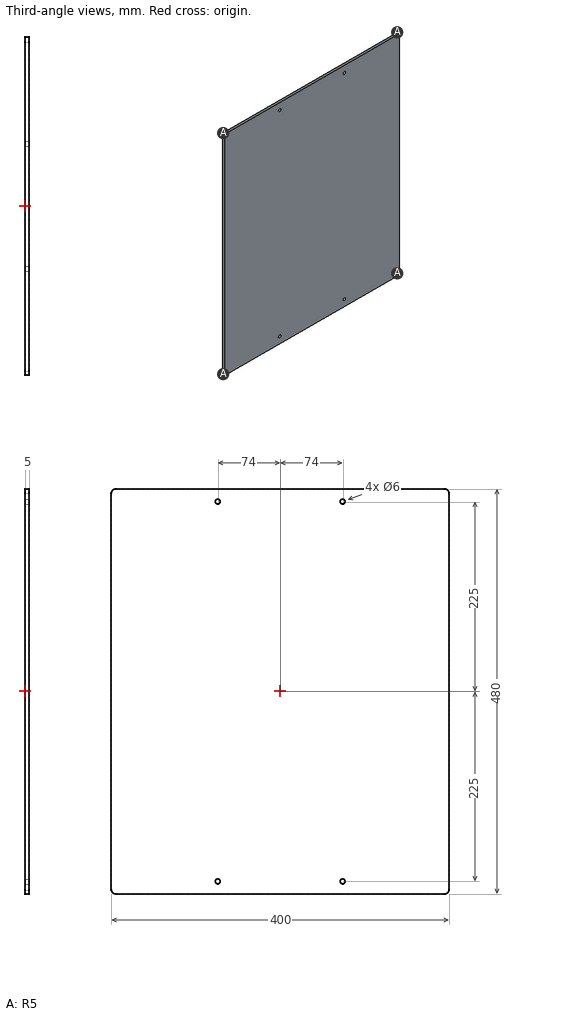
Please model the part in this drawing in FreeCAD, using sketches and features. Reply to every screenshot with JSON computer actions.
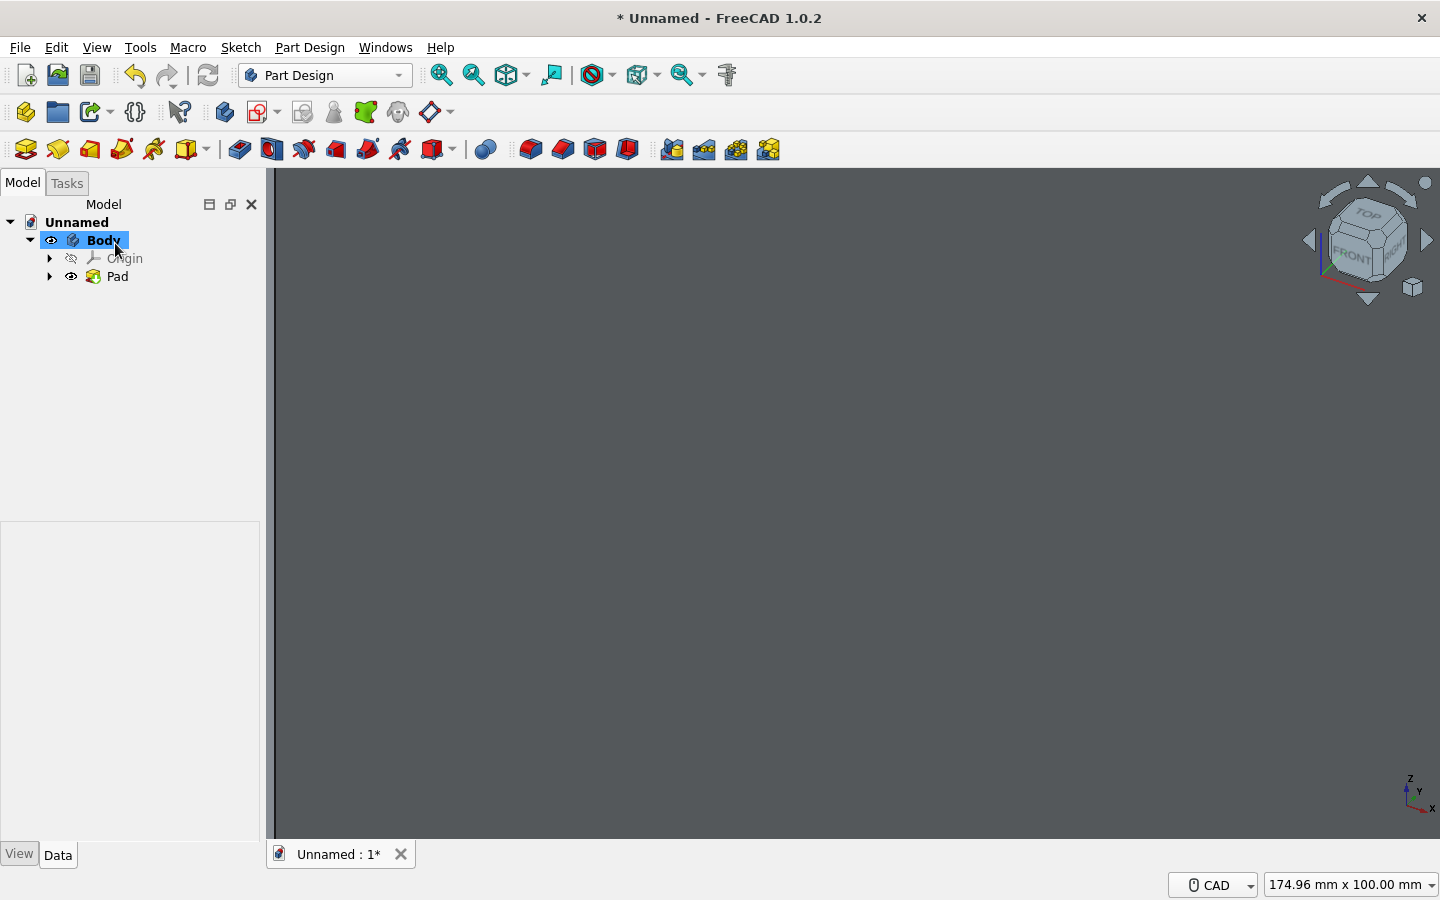
{"action": "left_click", "coordinate": [442, 76]}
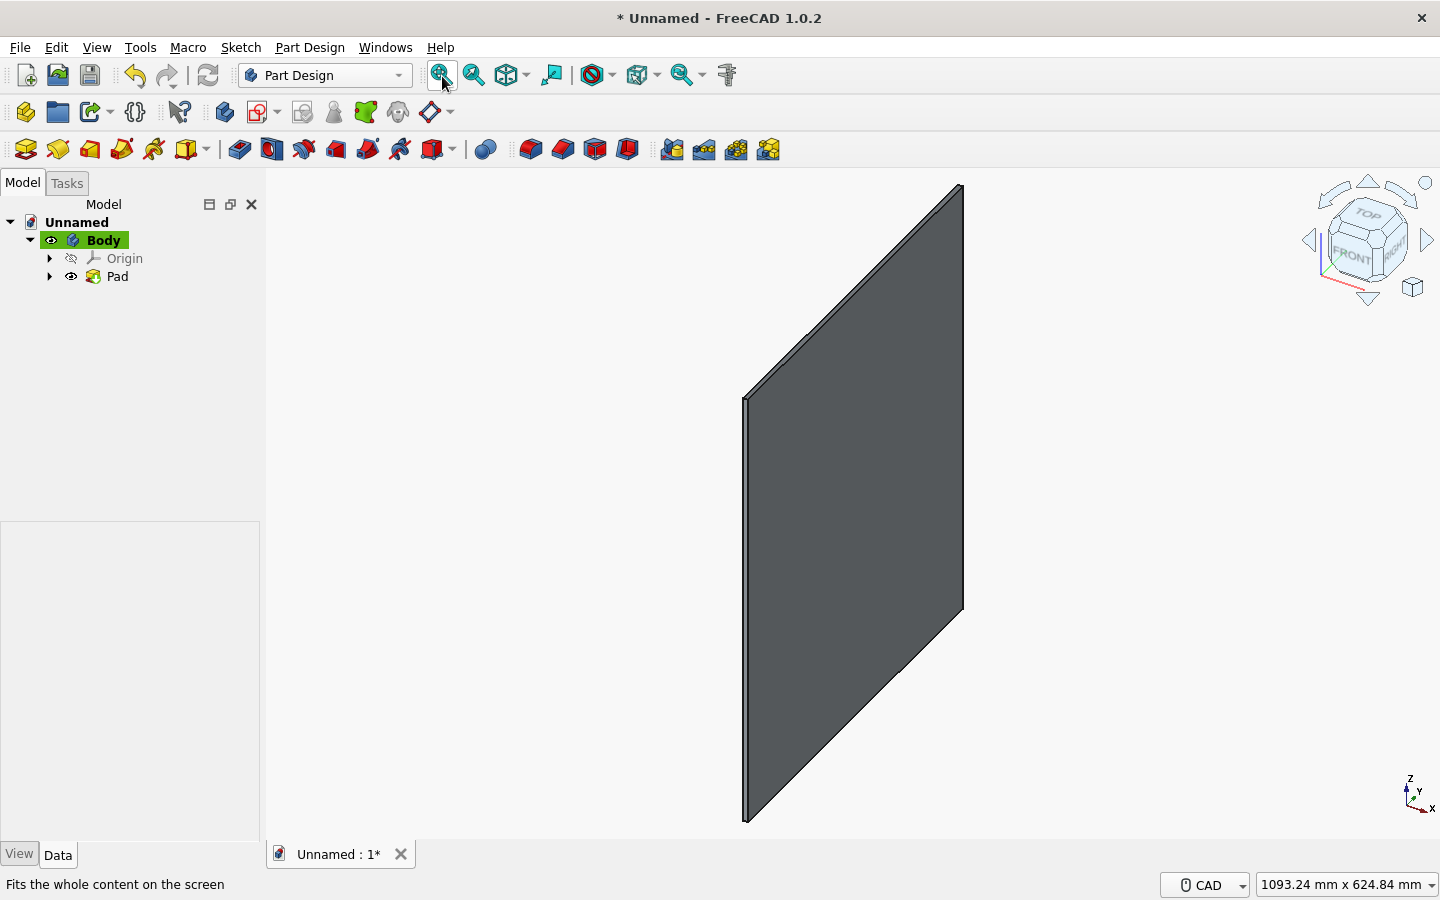
{"action": "left_click", "coordinate": [855, 503]}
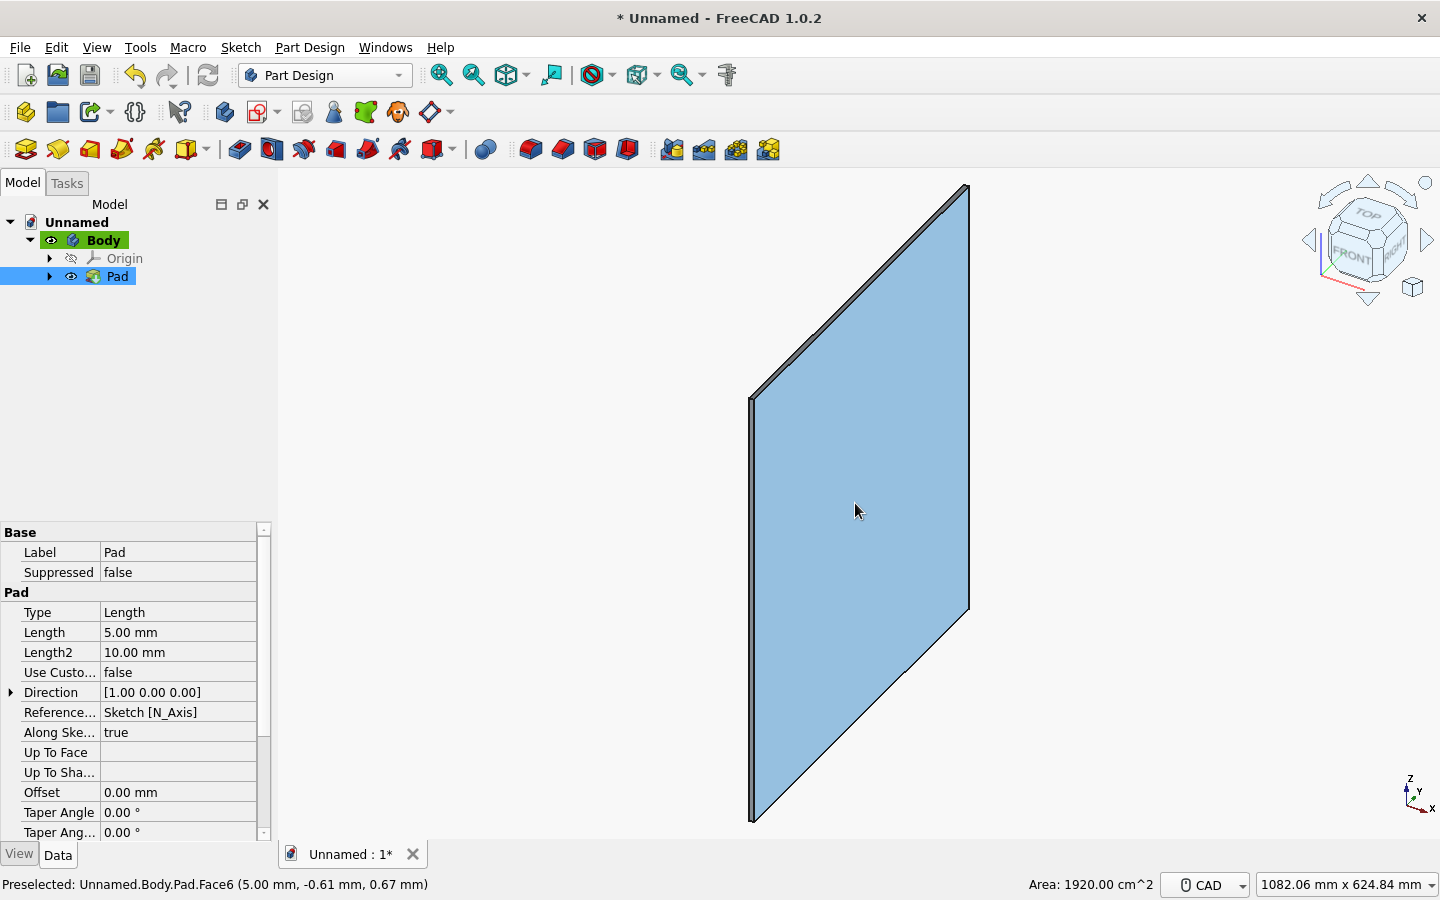
{"action": "left_click", "coordinate": [258, 112]}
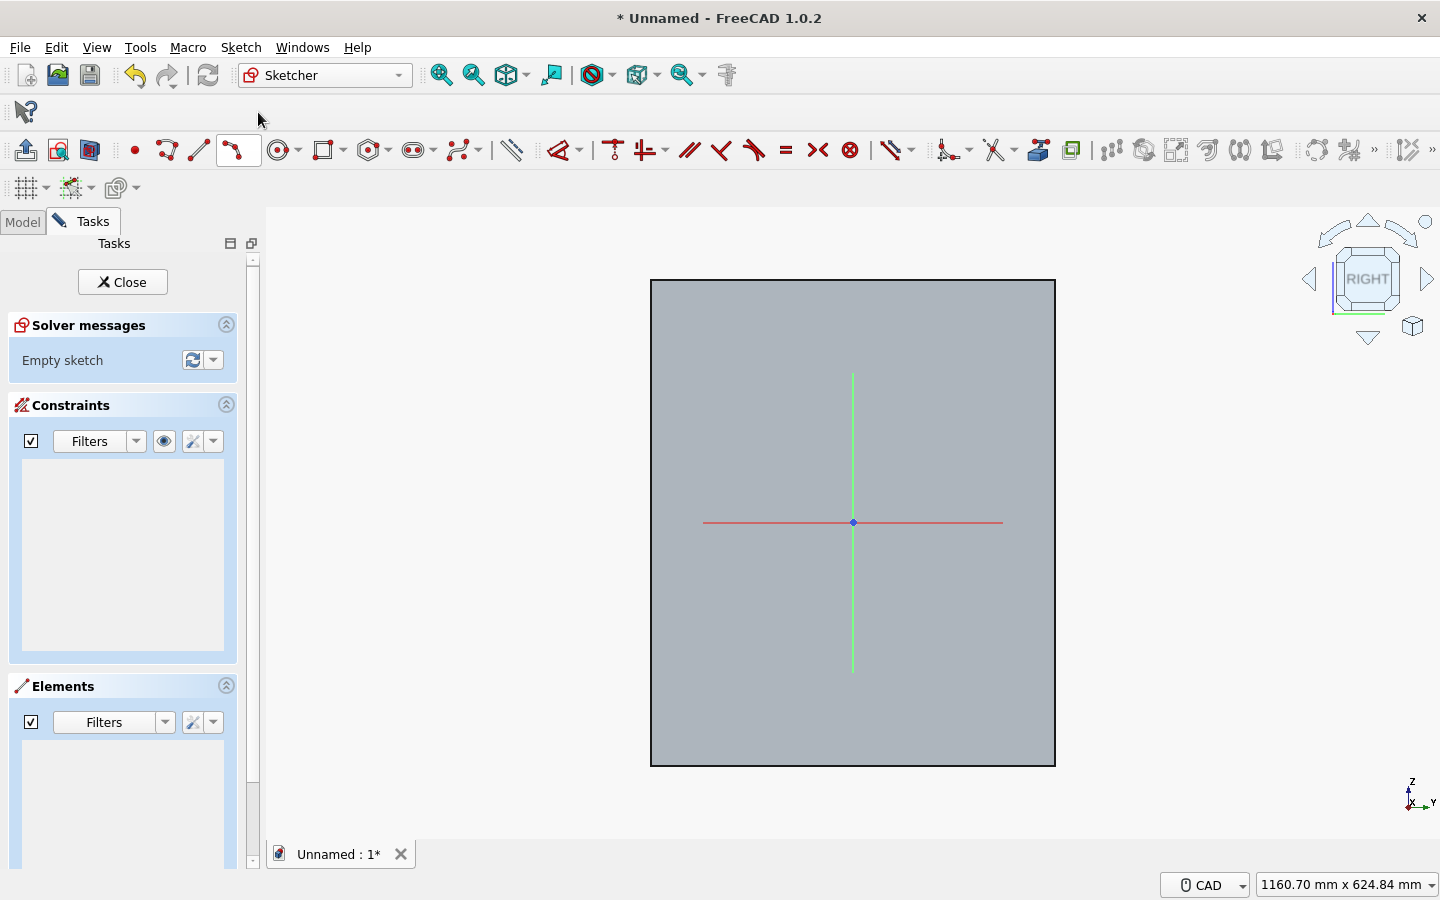
{"action": "left_click", "coordinate": [278, 150]}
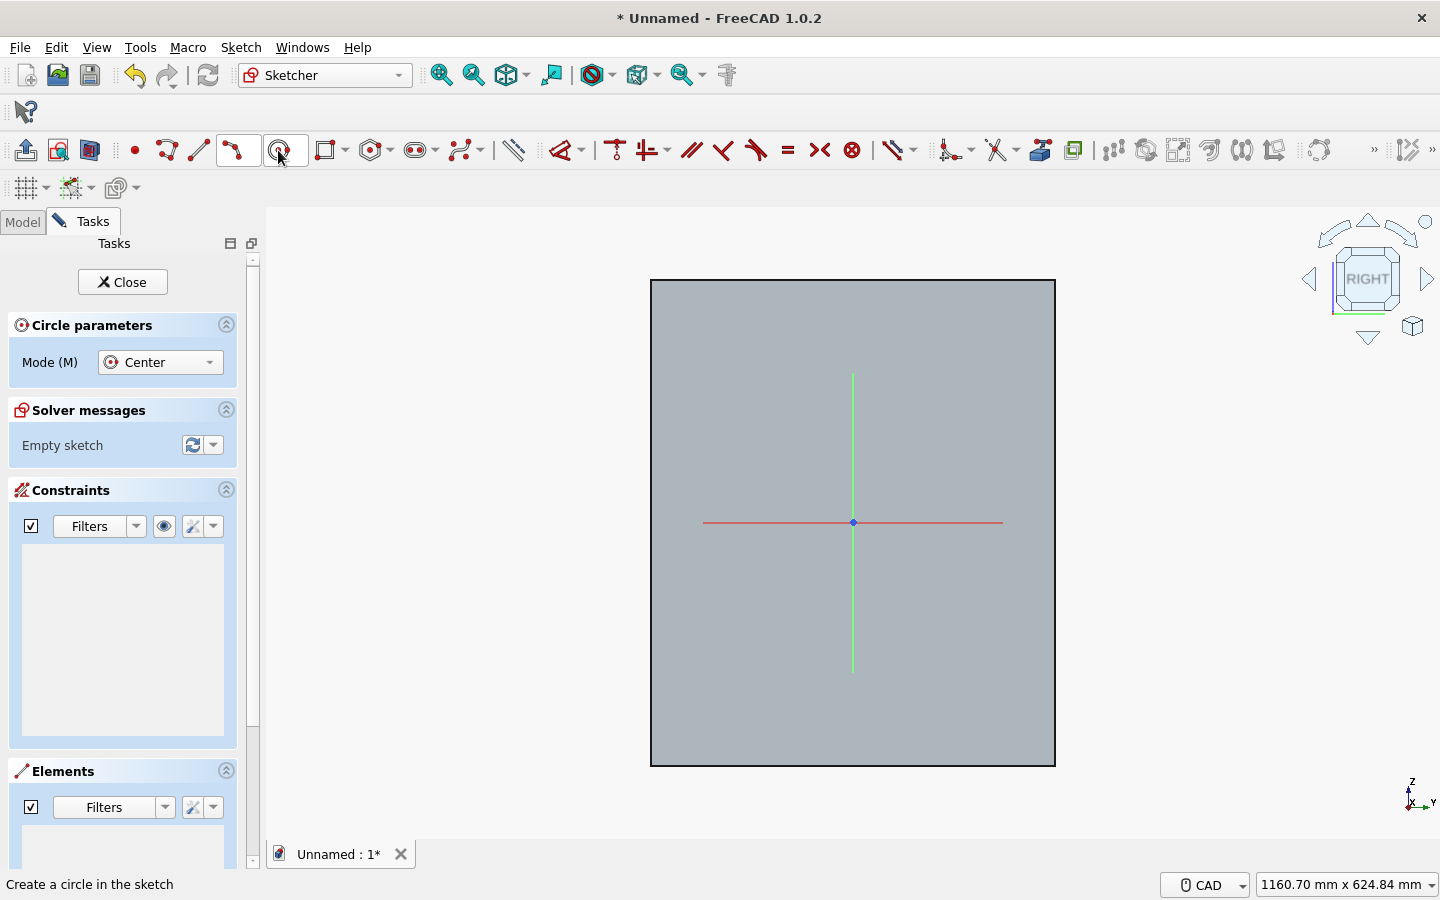
{"action": "scroll", "coordinate": [928, 295], "scroll_direction": "up", "scroll_amount": 11}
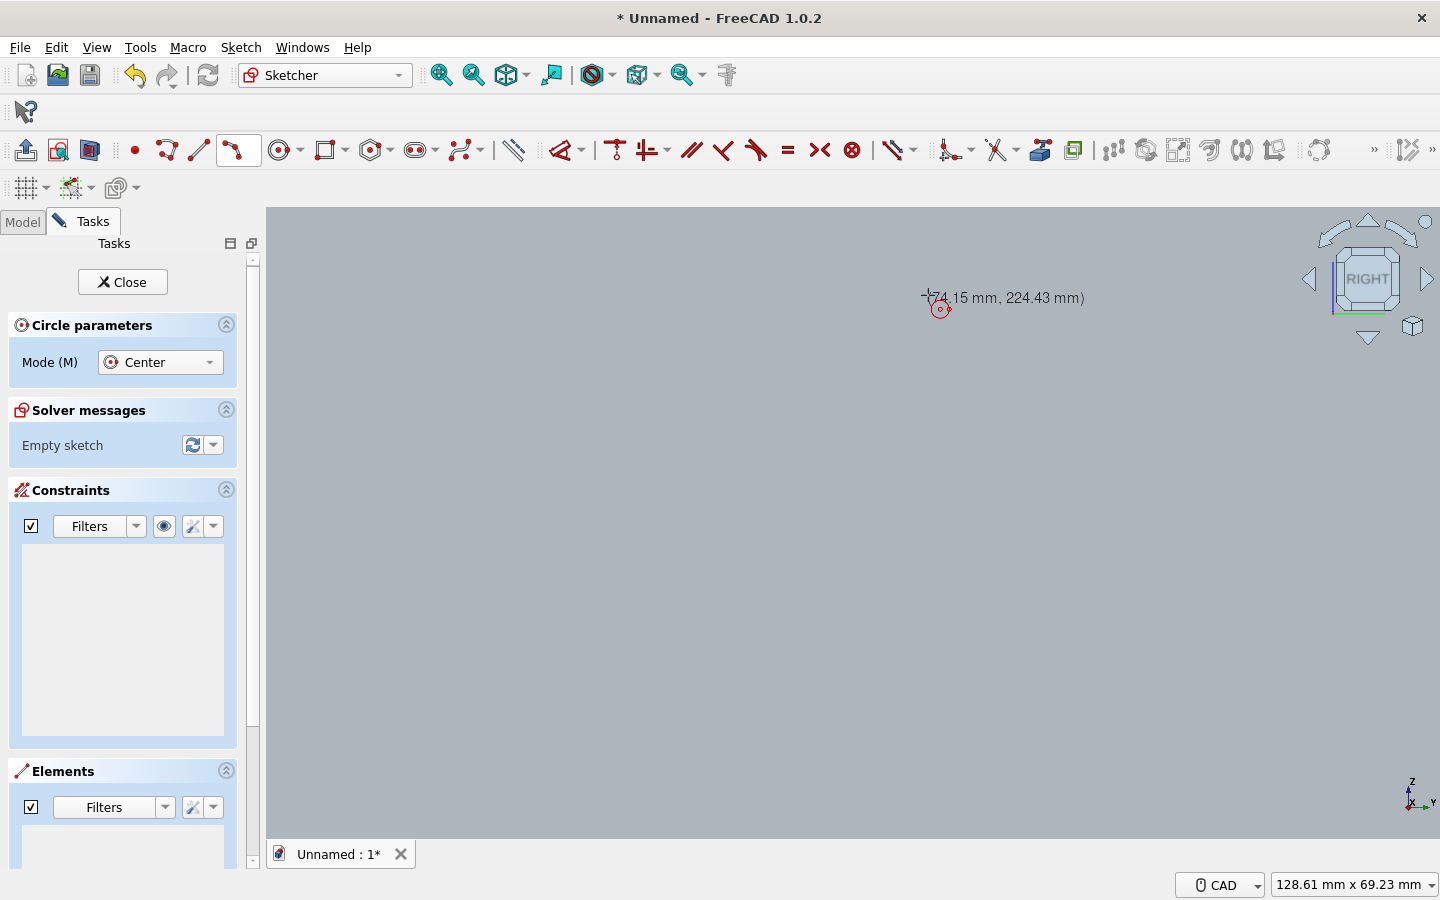
{"action": "scroll", "coordinate": [838, 341], "scroll_direction": "down", "scroll_amount": 12}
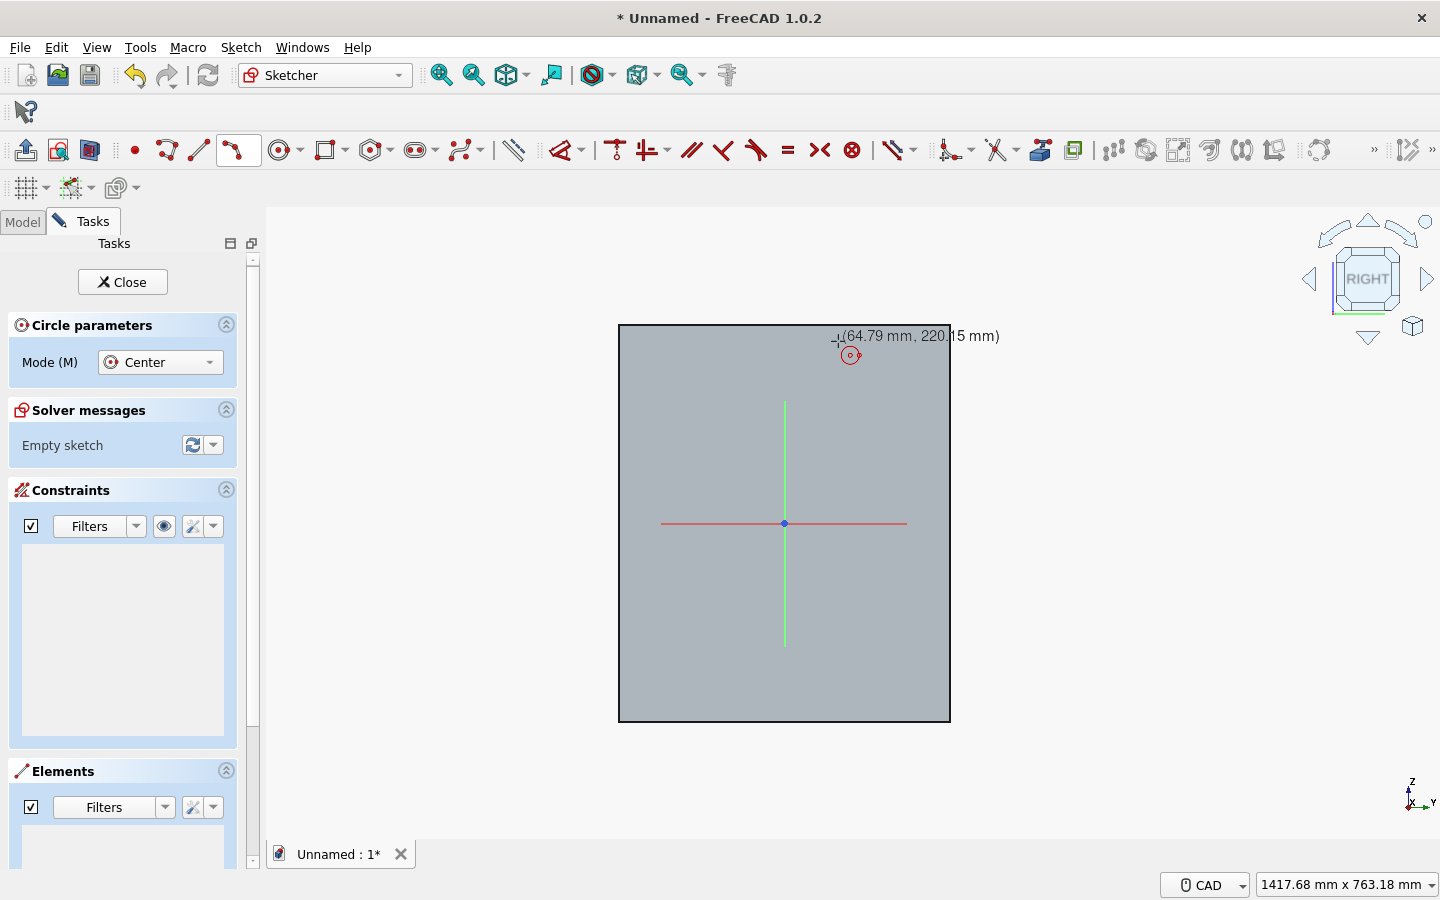
{"action": "left_click", "coordinate": [846, 337]}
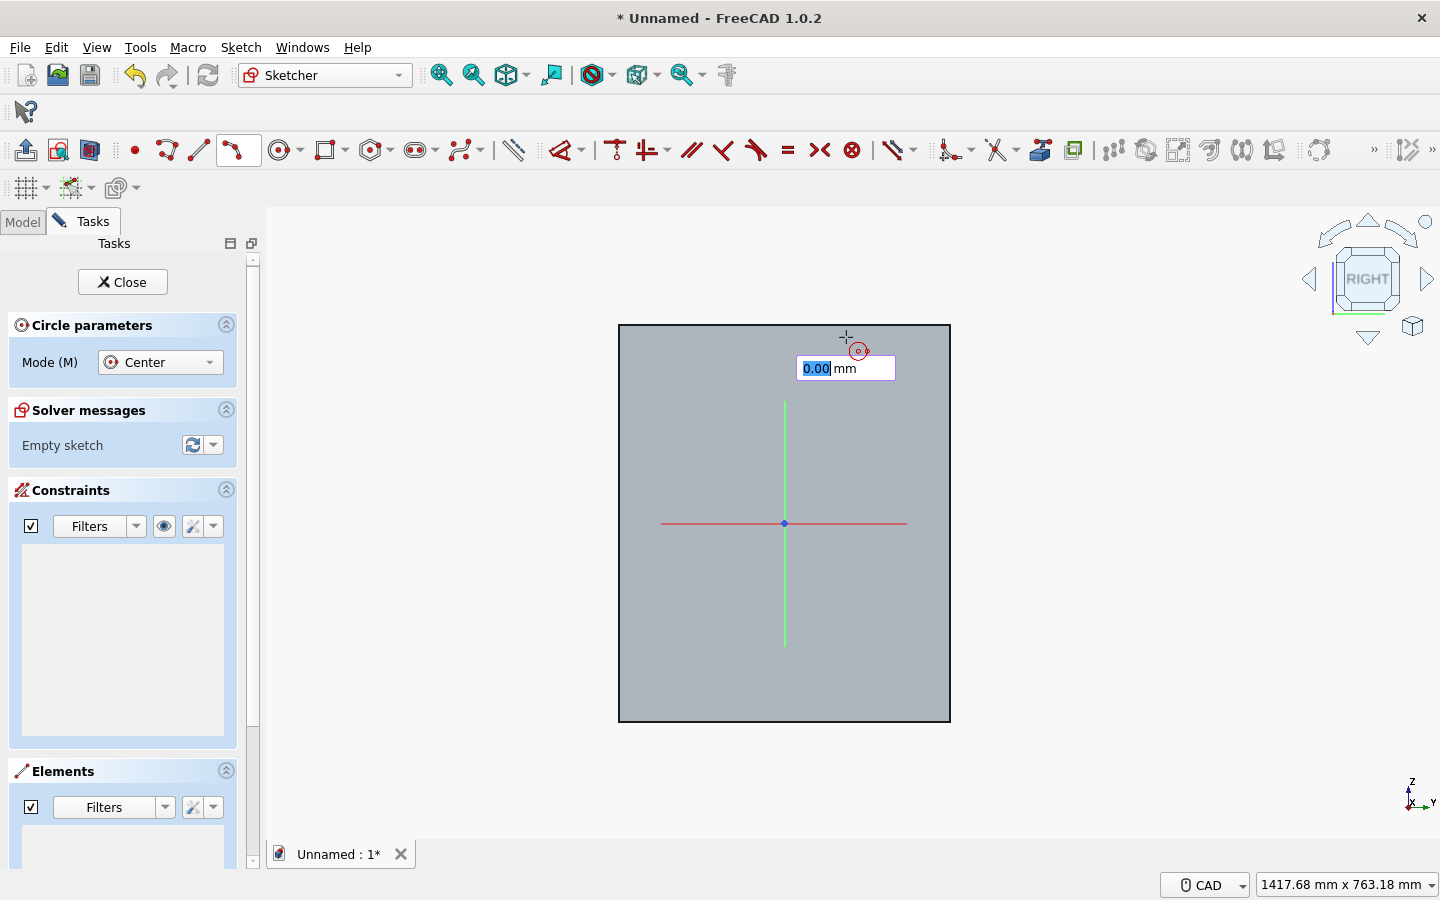
{"action": "scroll", "coordinate": [848, 336], "scroll_direction": "up", "scroll_amount": 10}